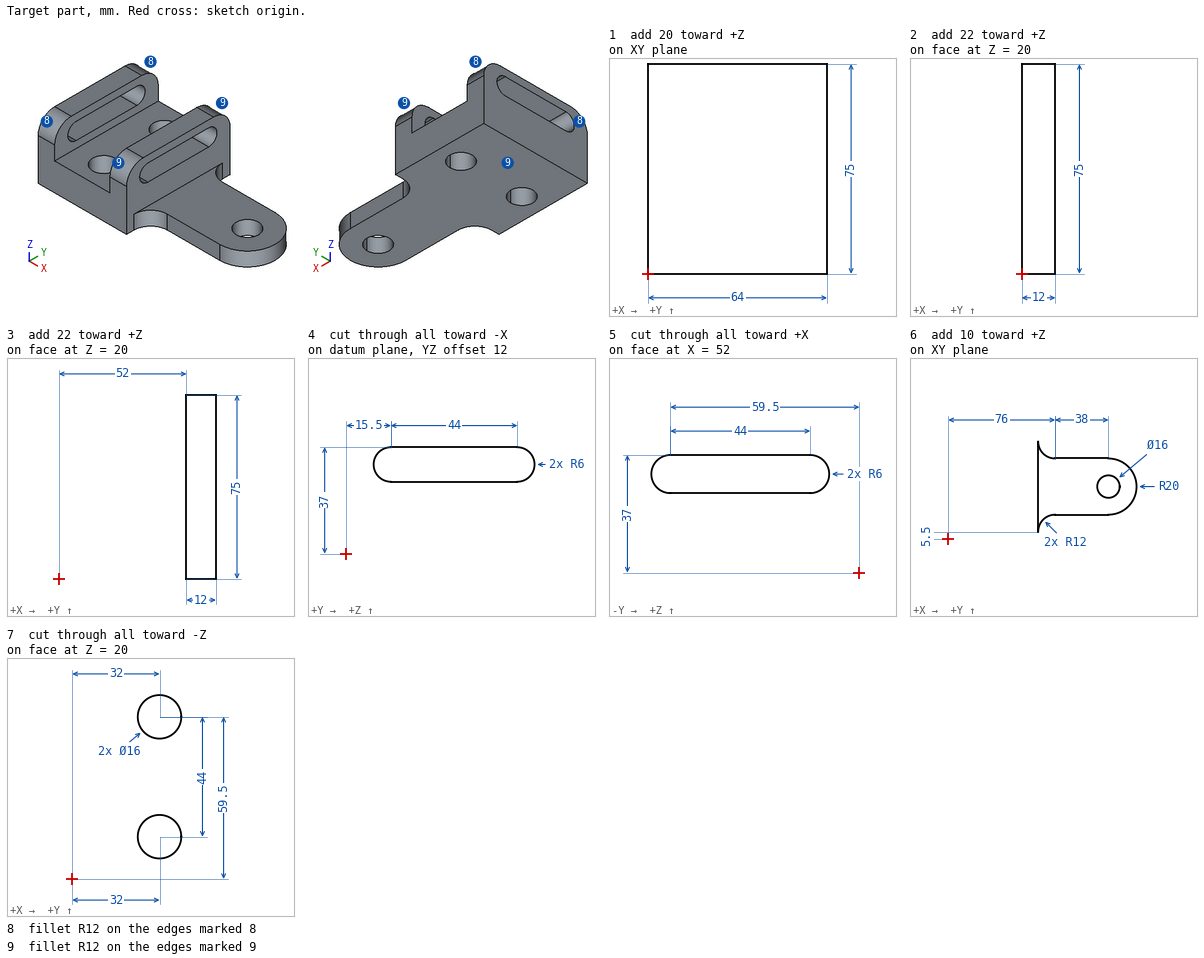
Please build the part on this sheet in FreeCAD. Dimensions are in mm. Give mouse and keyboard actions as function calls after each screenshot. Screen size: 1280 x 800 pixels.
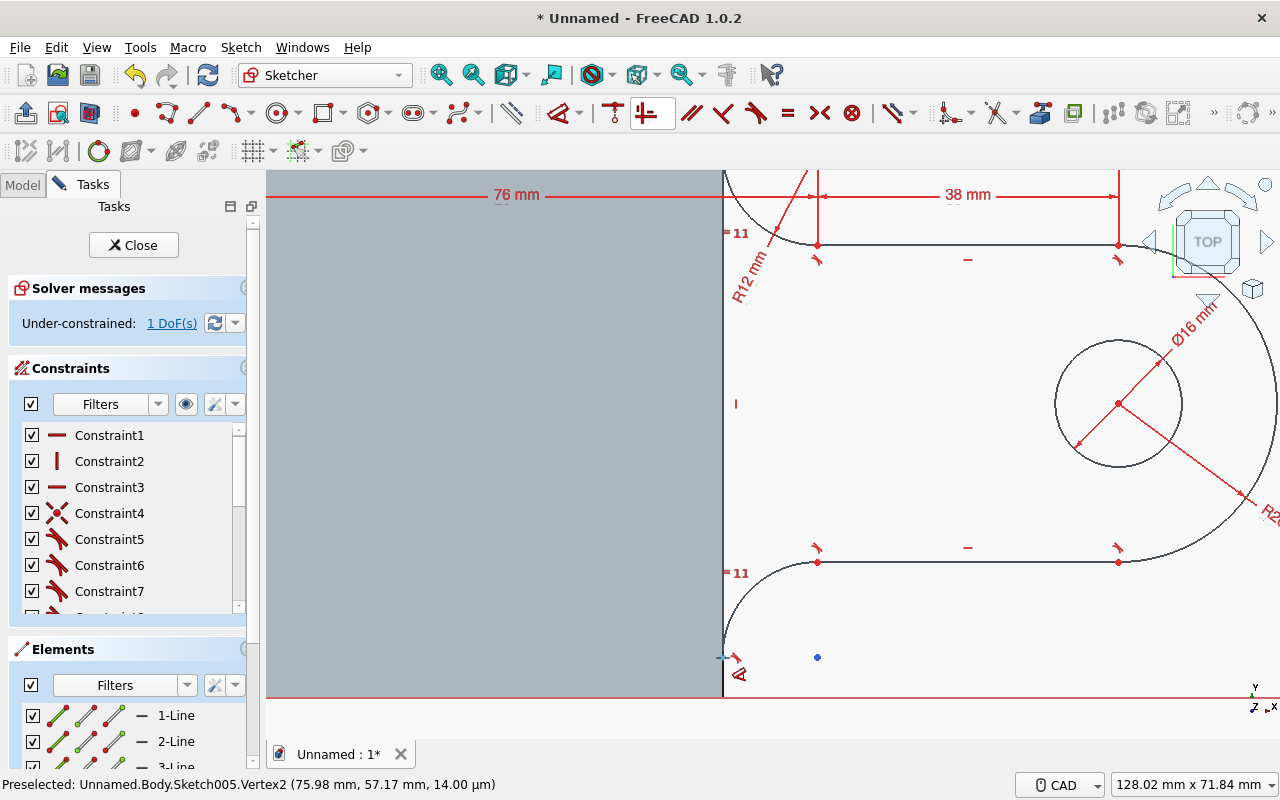
click(723, 657)
click(757, 678)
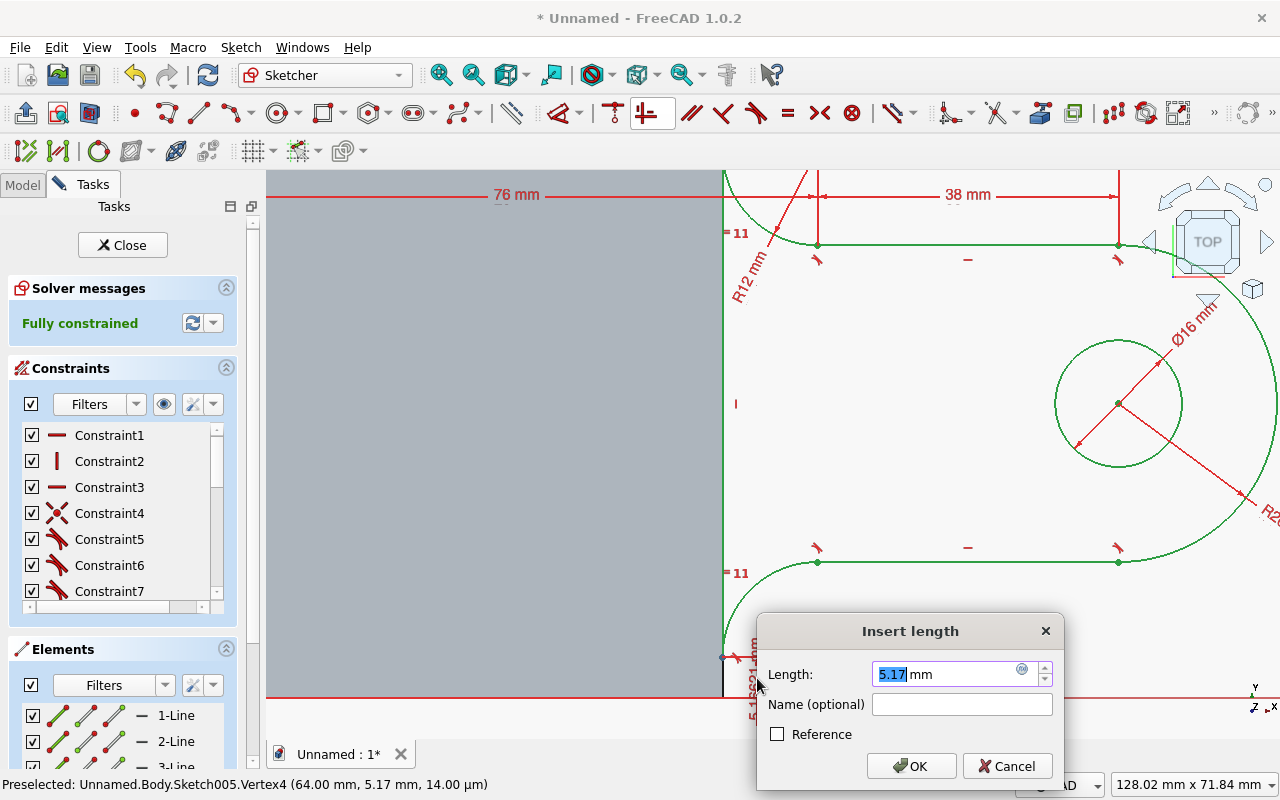
text(5.5)
key(Return)
key(Escape)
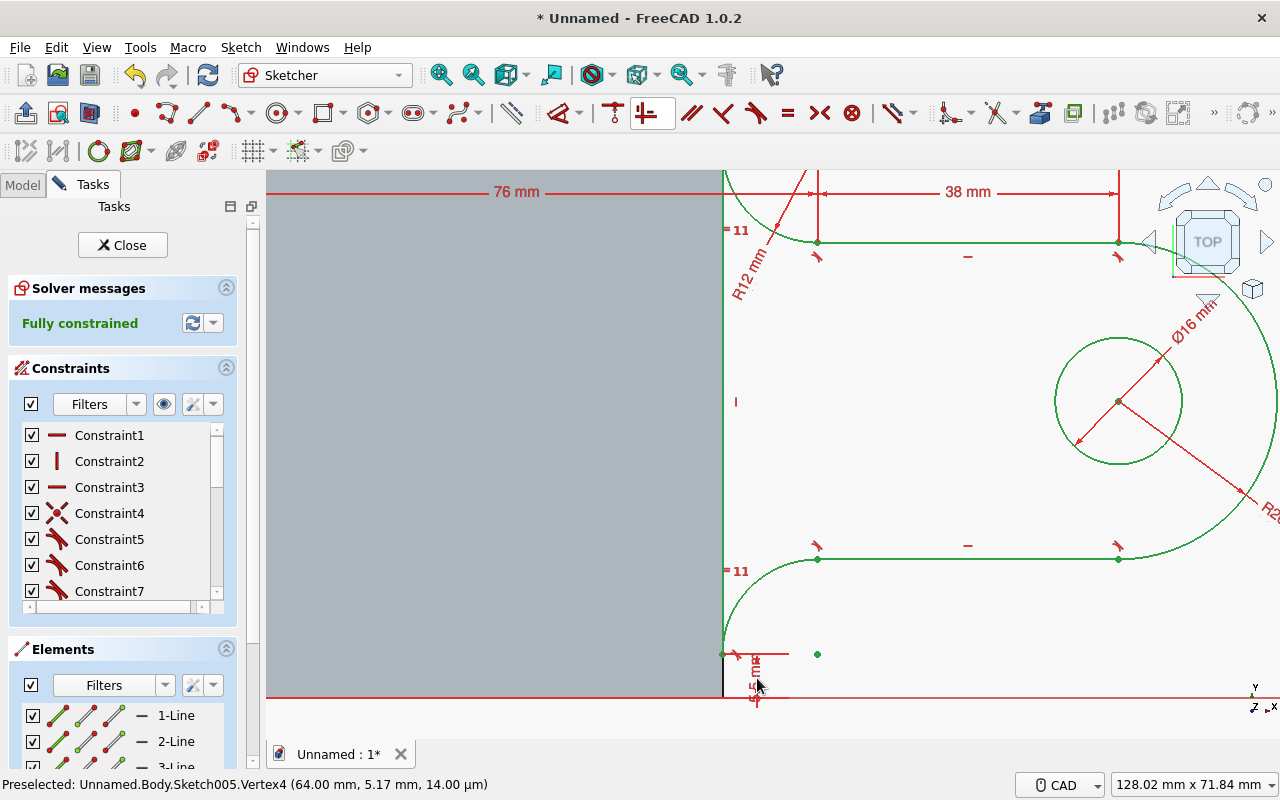
click(123, 245)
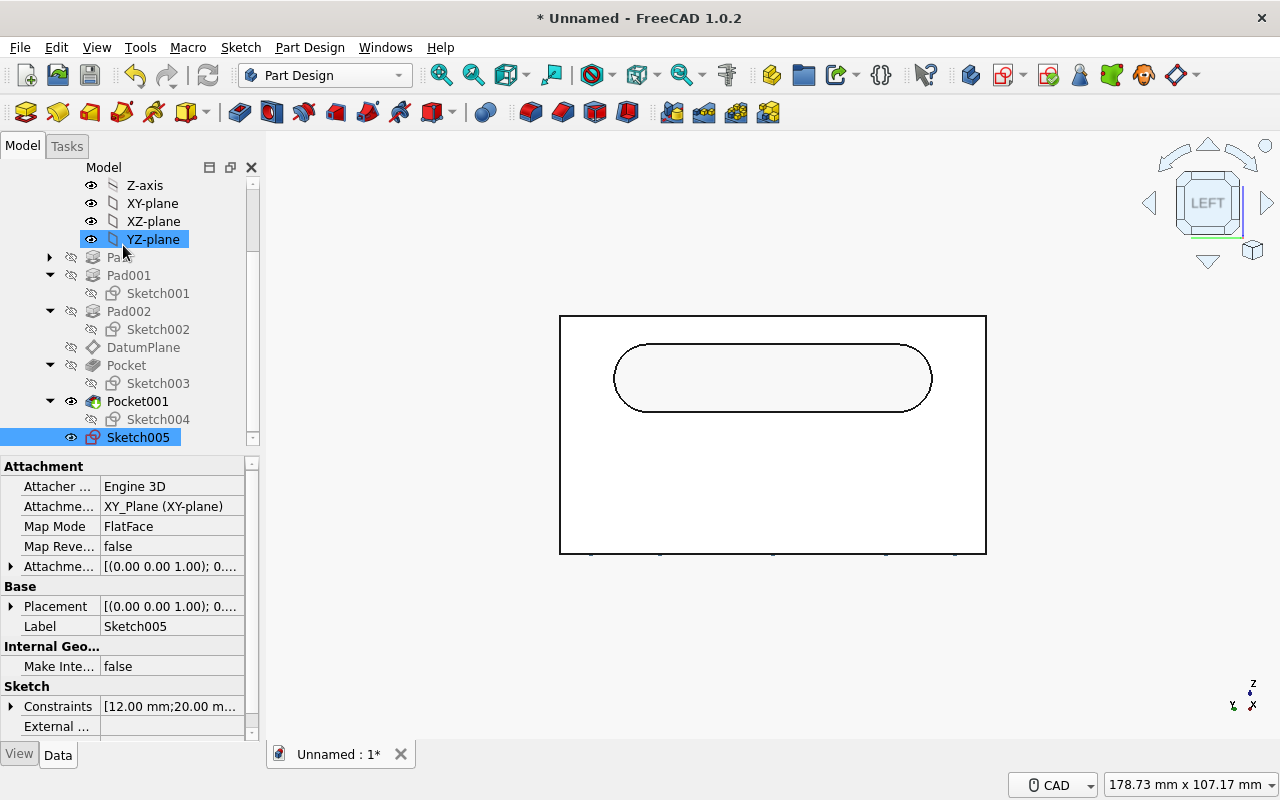
click(26, 112)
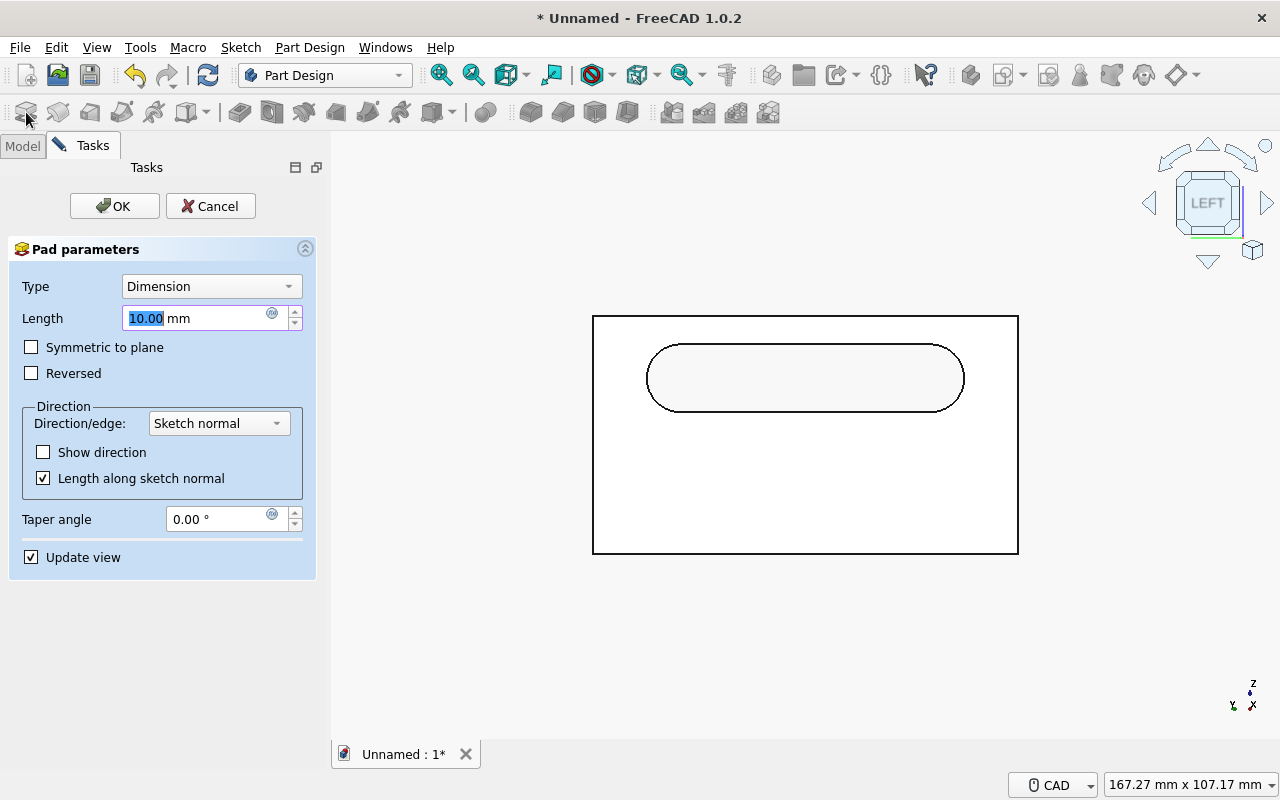
text(10)
key(Tab)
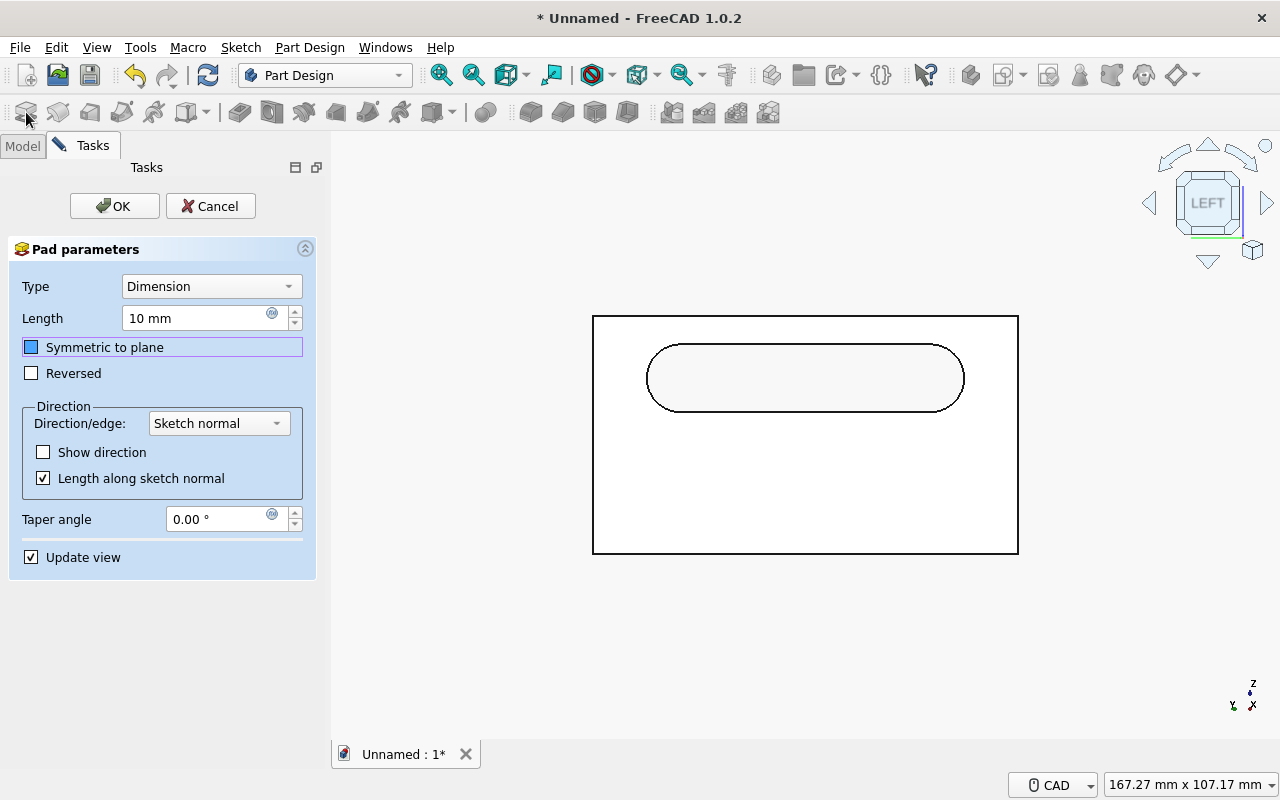
click(115, 206)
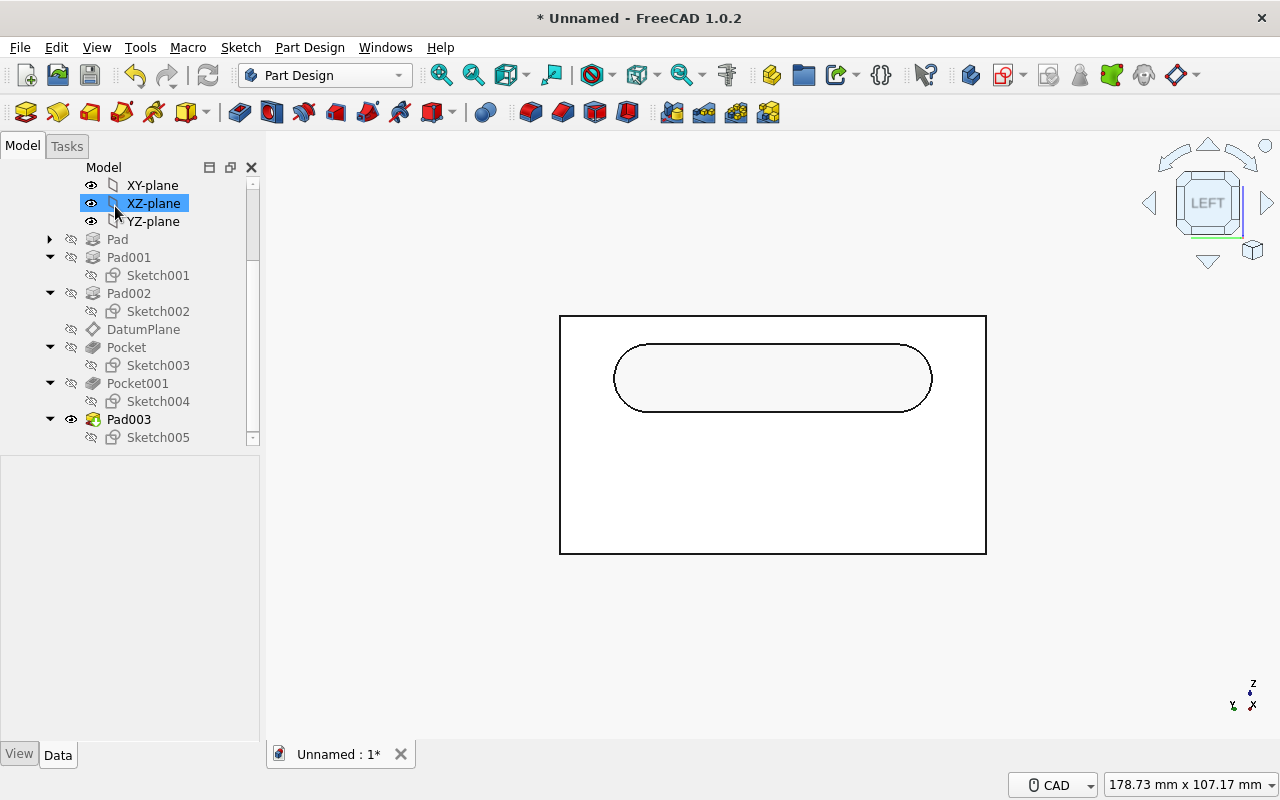
click(442, 76)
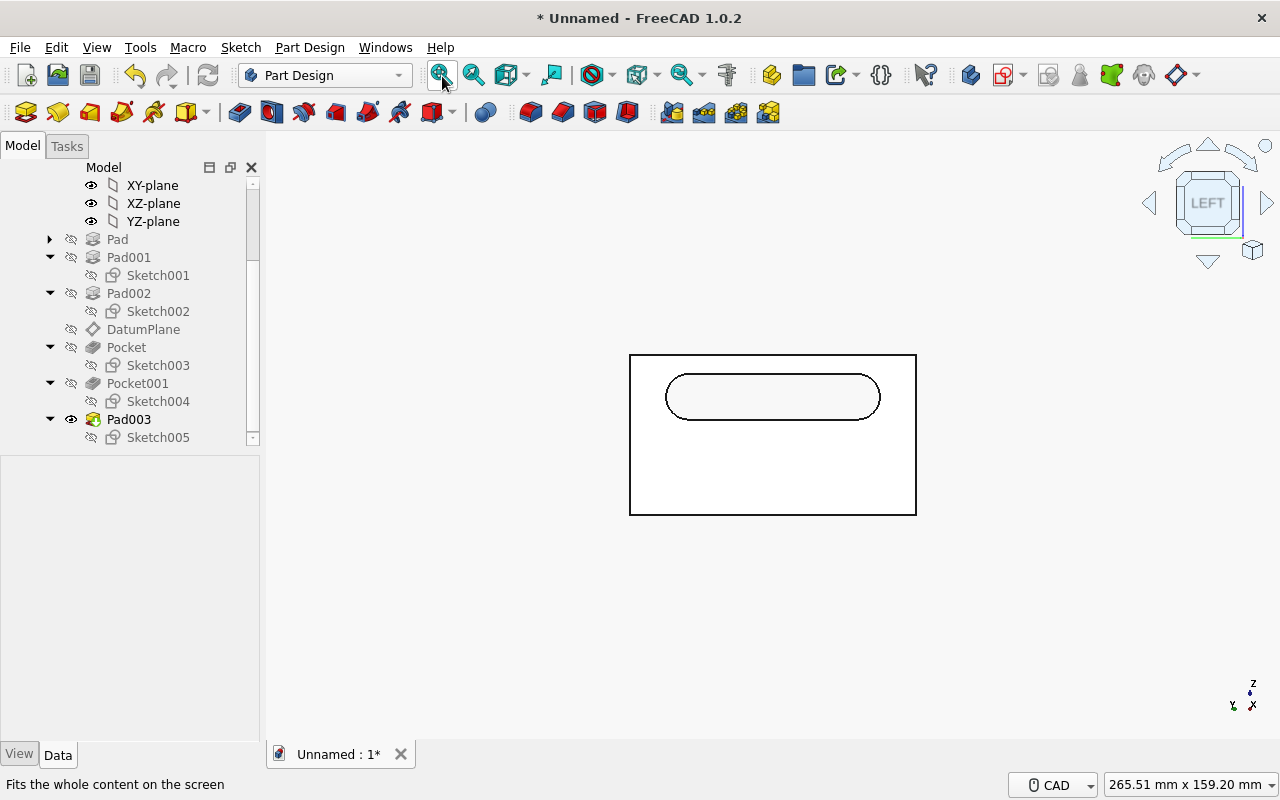
key(0)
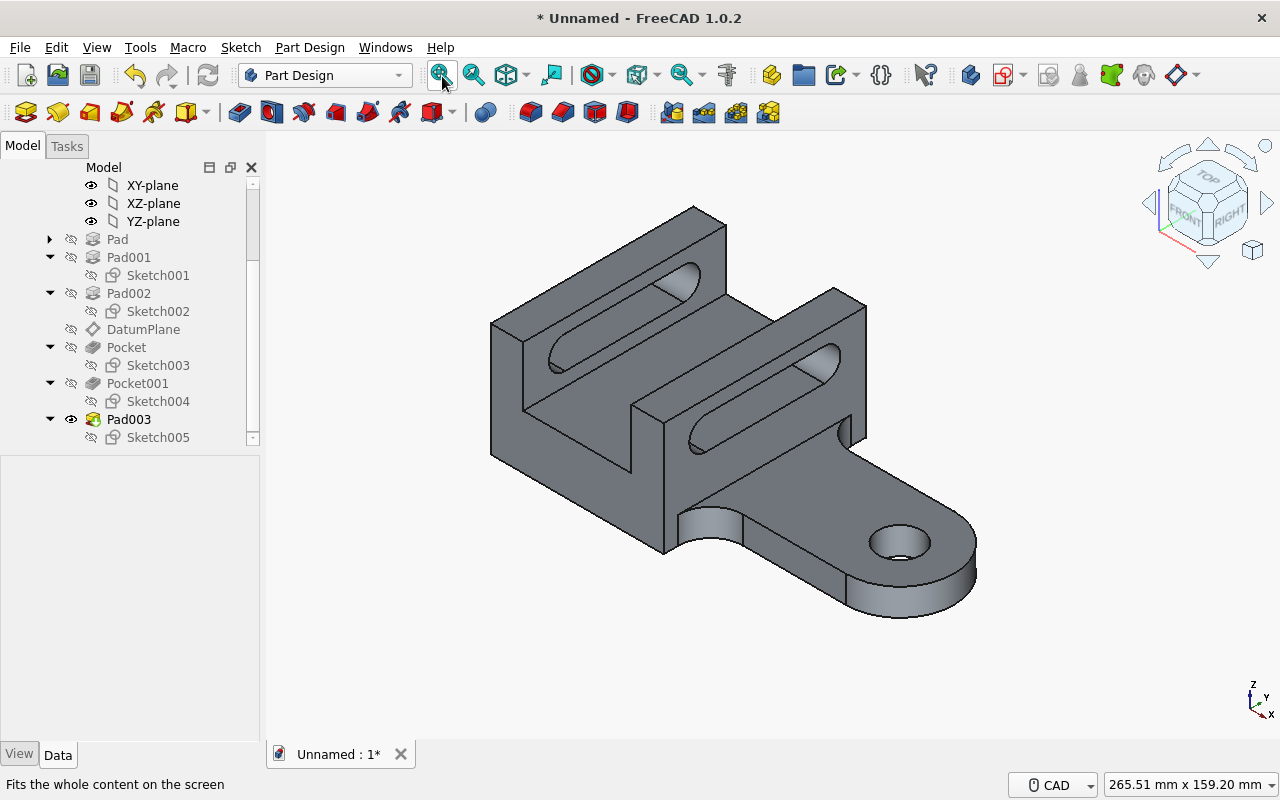
click(621, 416)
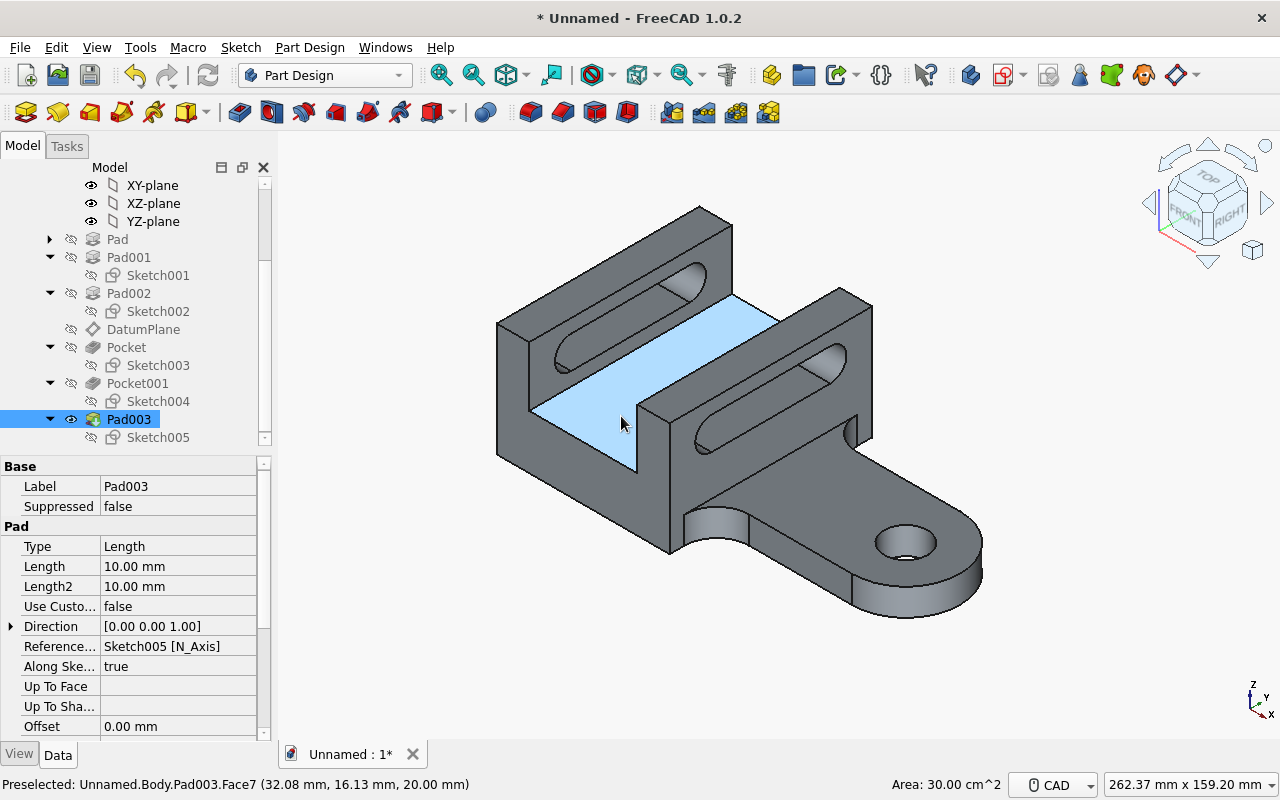
click(1004, 76)